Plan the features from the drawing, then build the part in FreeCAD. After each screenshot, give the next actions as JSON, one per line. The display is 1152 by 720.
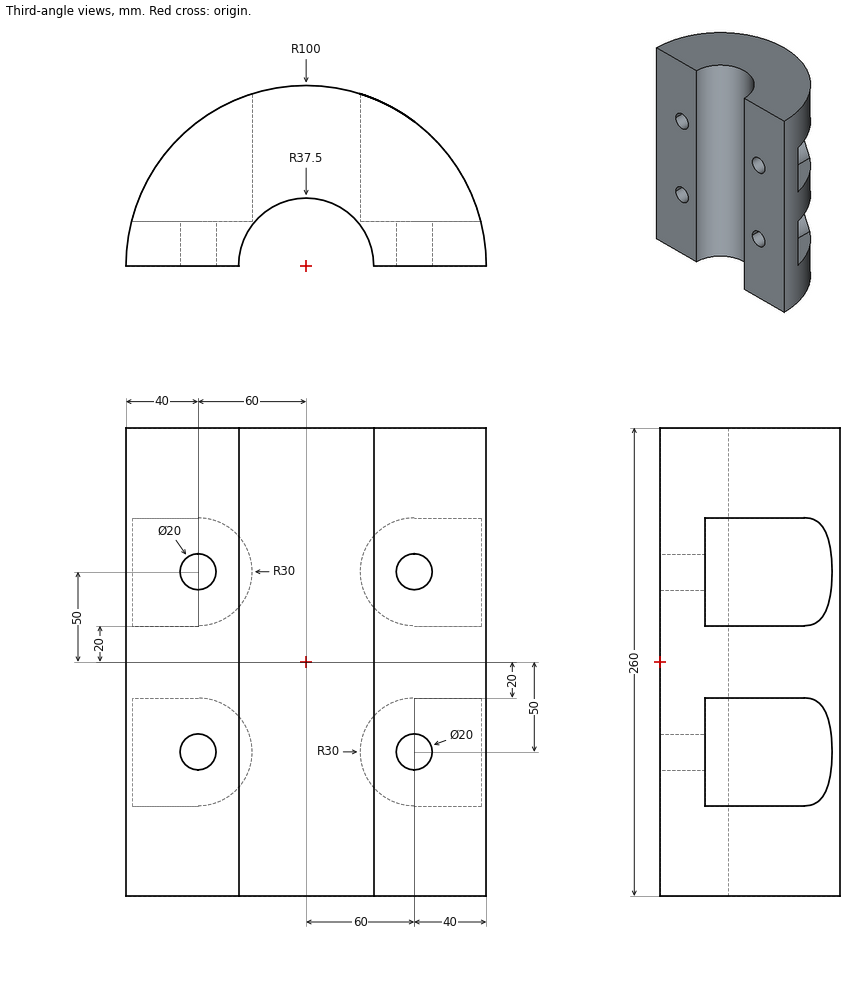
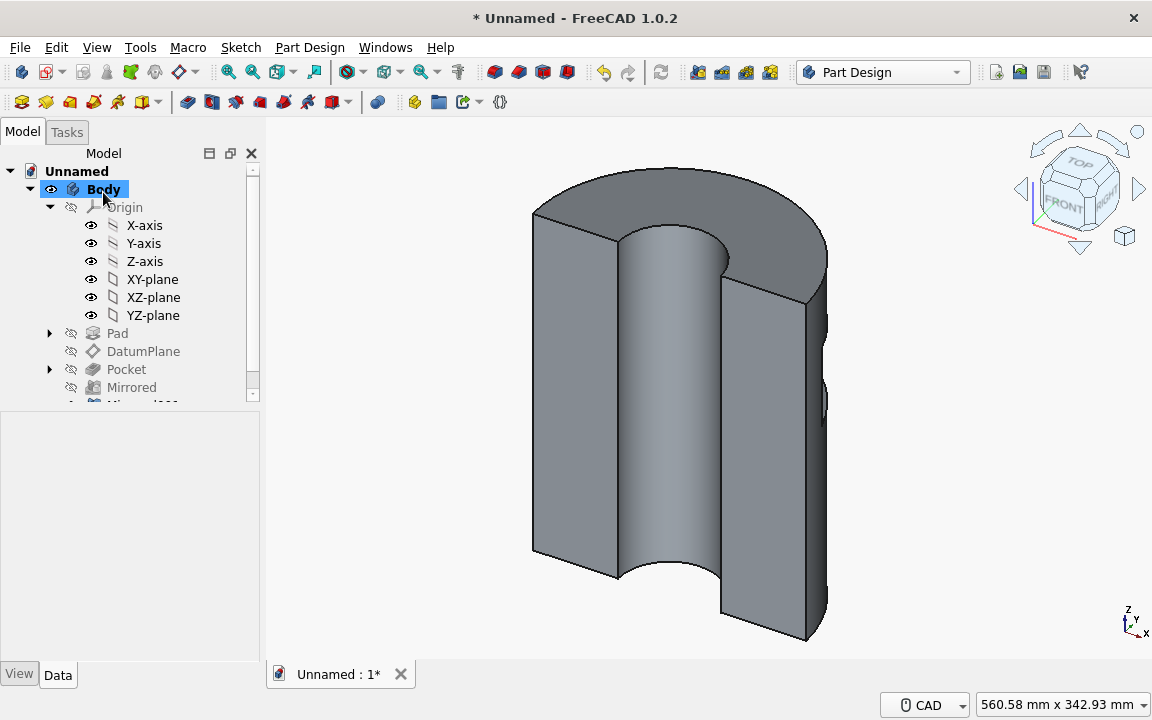
{"action": "key", "text": "4"}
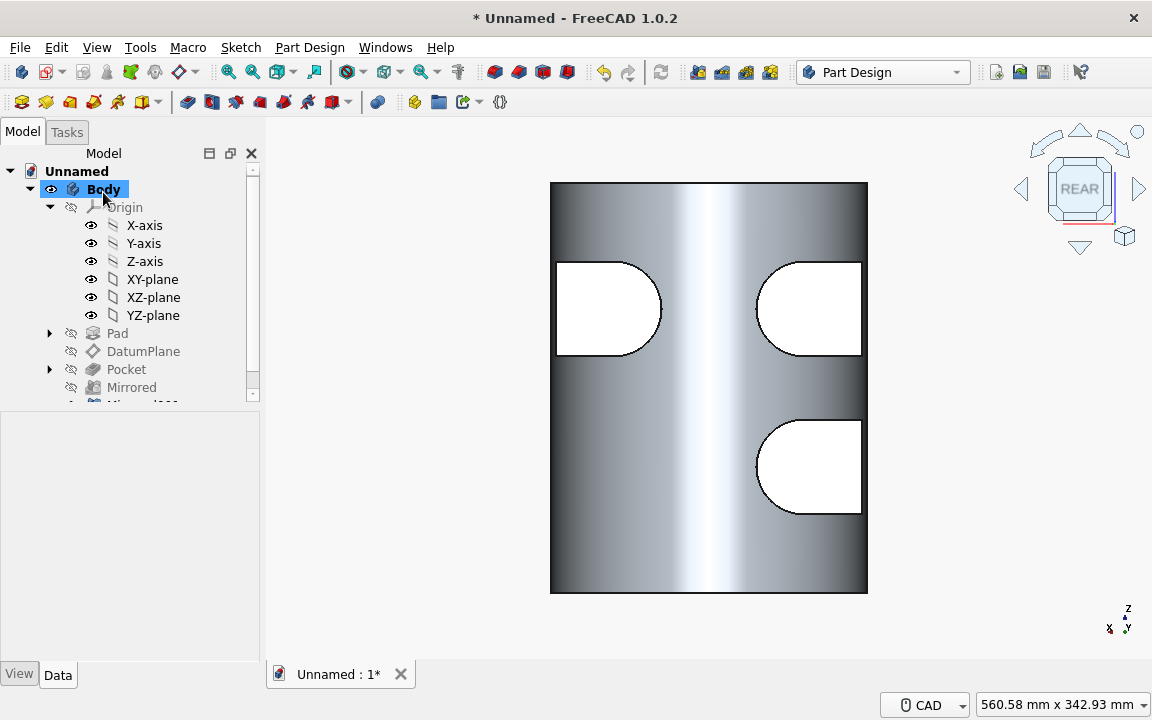
{"action": "left_click", "coordinate": [609, 308]}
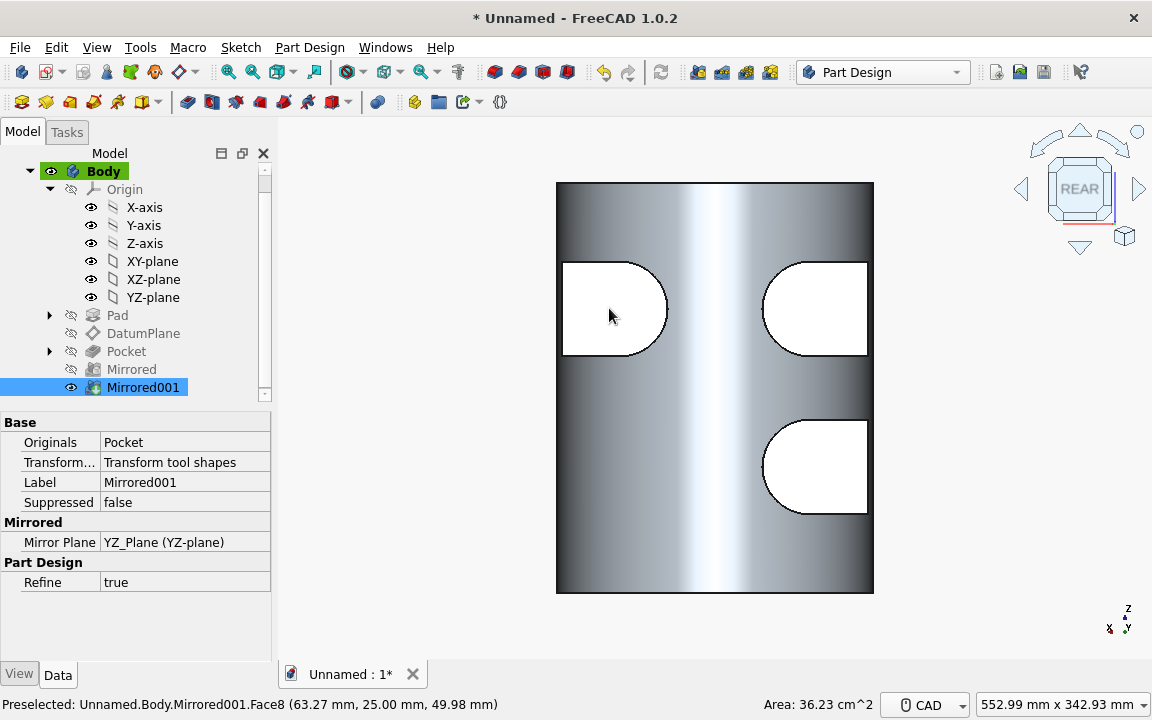
{"action": "left_click", "coordinate": [46, 72]}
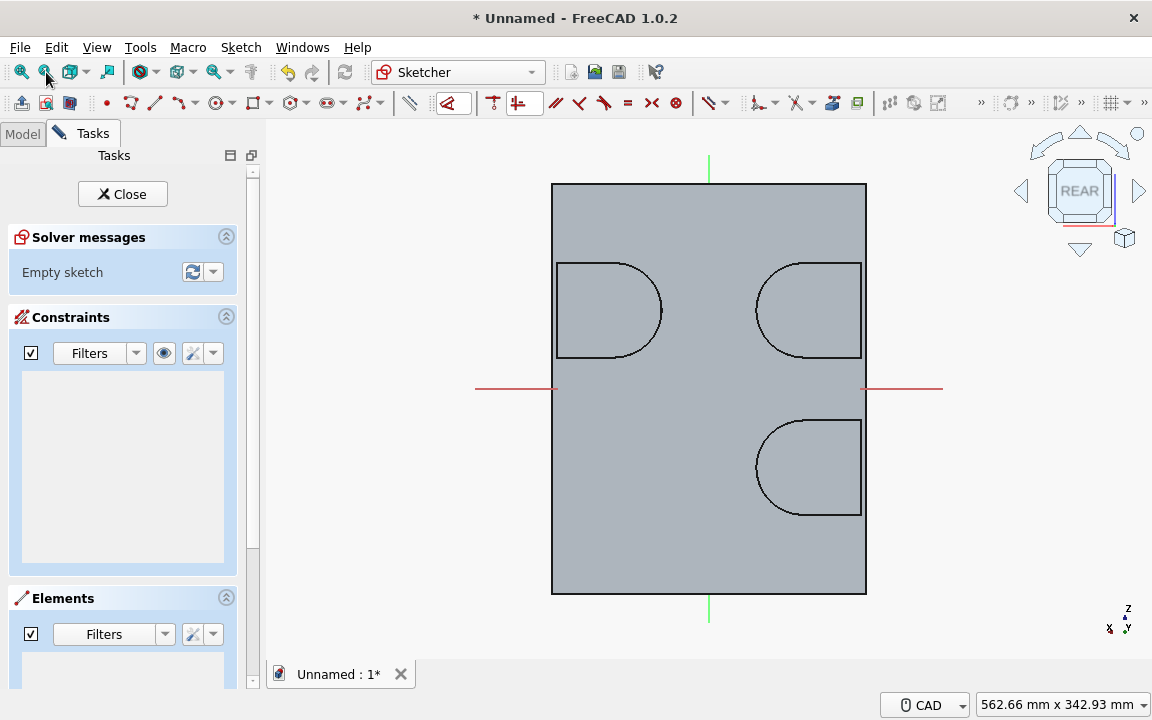
{"action": "scroll", "coordinate": [624, 489], "scroll_direction": "up", "scroll_amount": 5}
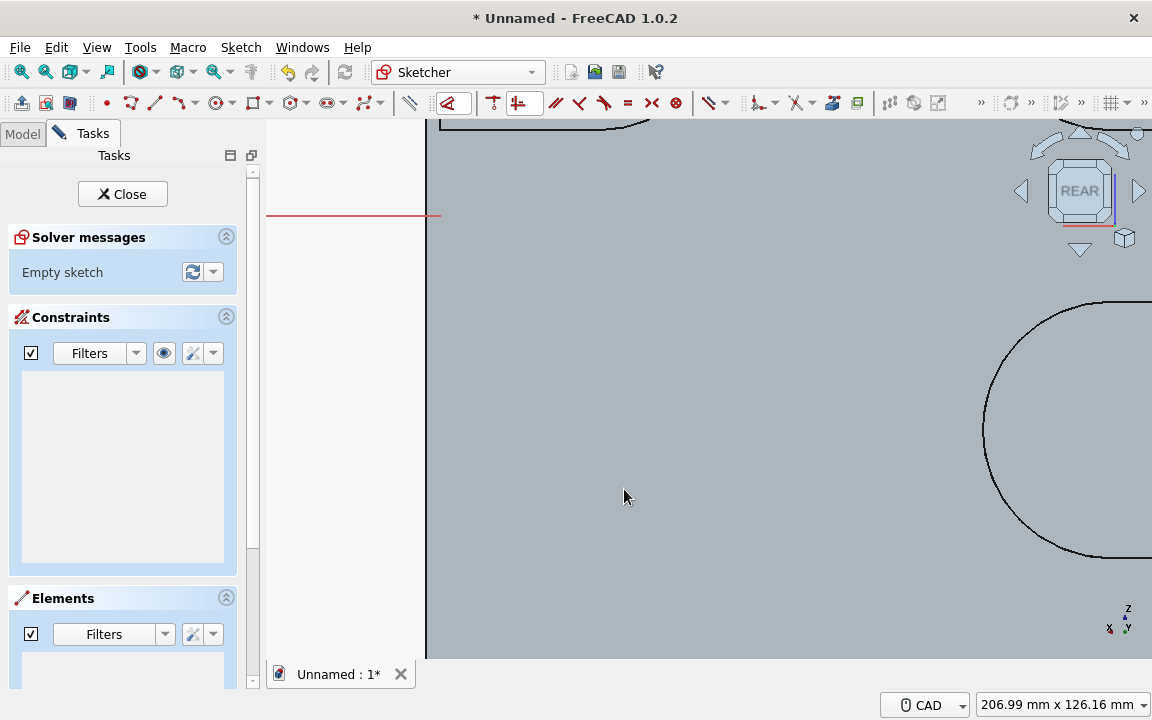
{"action": "left_click", "coordinate": [132, 104]}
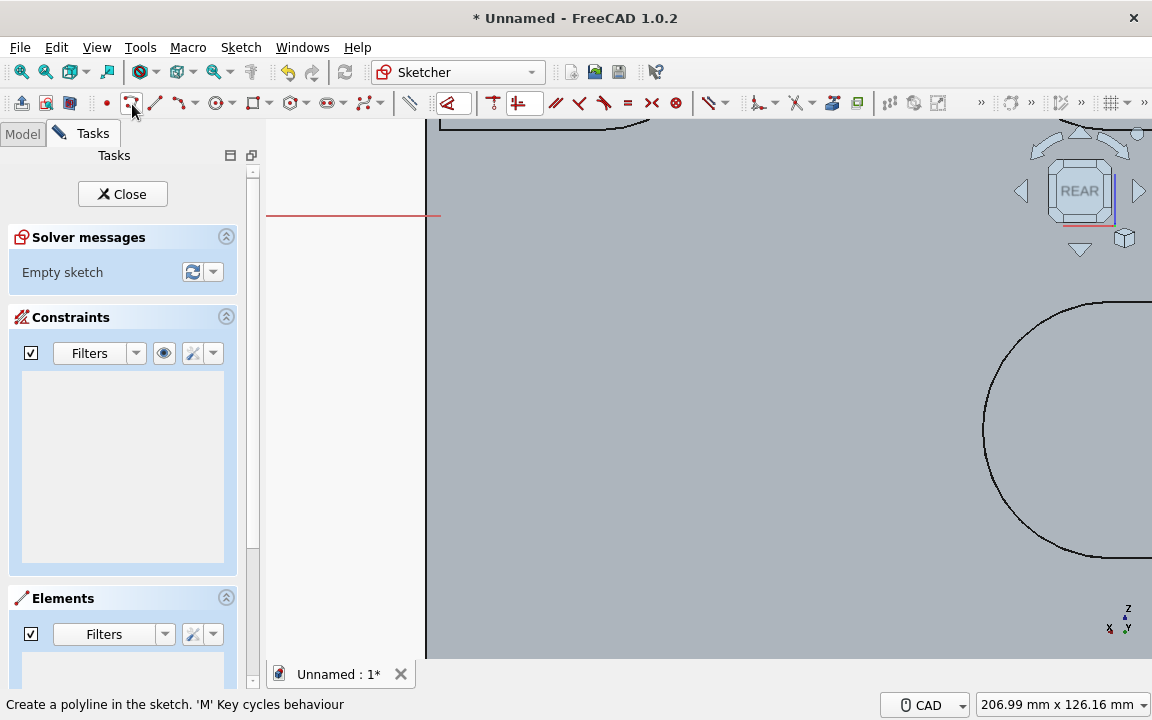
{"action": "left_click", "coordinate": [598, 302]}
{"action": "left_click", "coordinate": [426, 302]}
{"action": "left_click", "coordinate": [426, 558]}
{"action": "left_click", "coordinate": [598, 558]}
{"action": "right_click", "coordinate": [598, 558]}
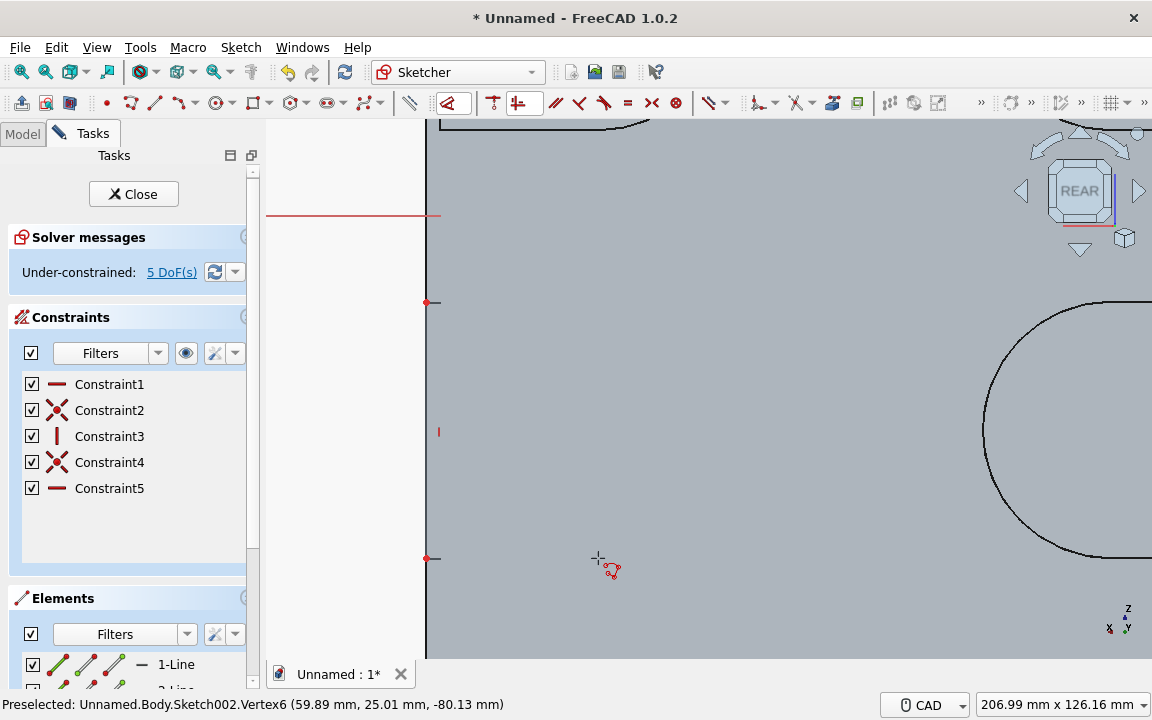
{"action": "key", "text": "g 3 a"}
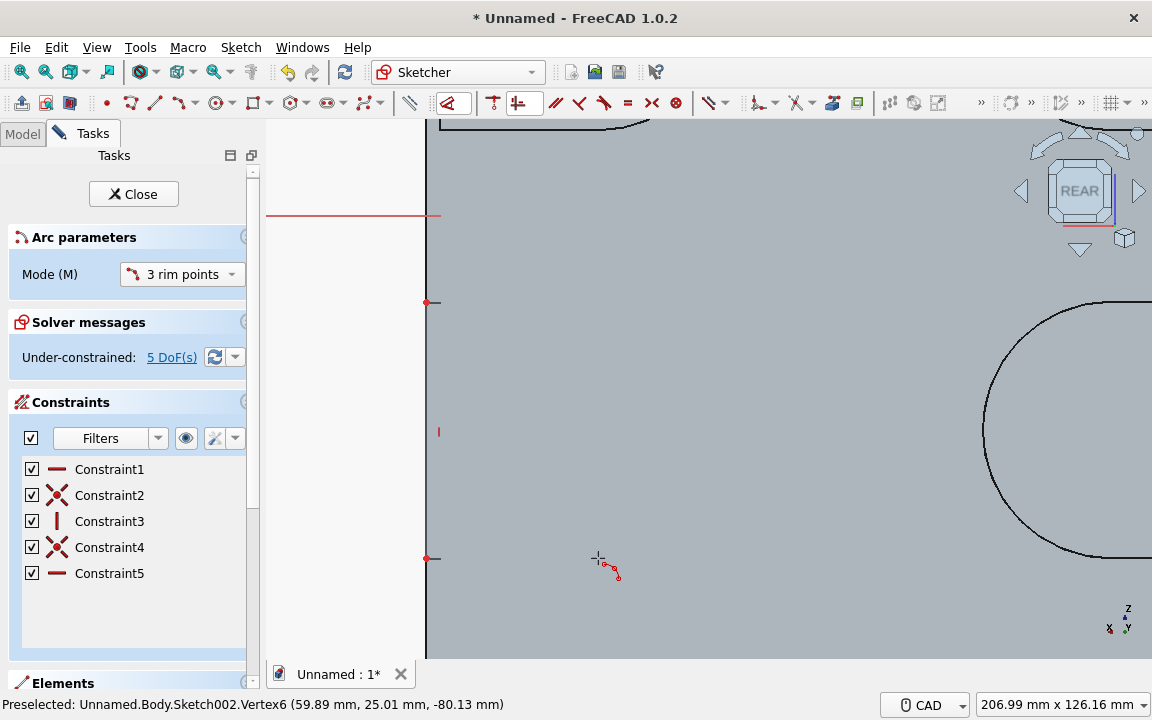
{"action": "left_click", "coordinate": [598, 559]}
{"action": "left_click", "coordinate": [598, 303]}
{"action": "left_click", "coordinate": [726, 430]}
{"action": "key", "text": "Escape"}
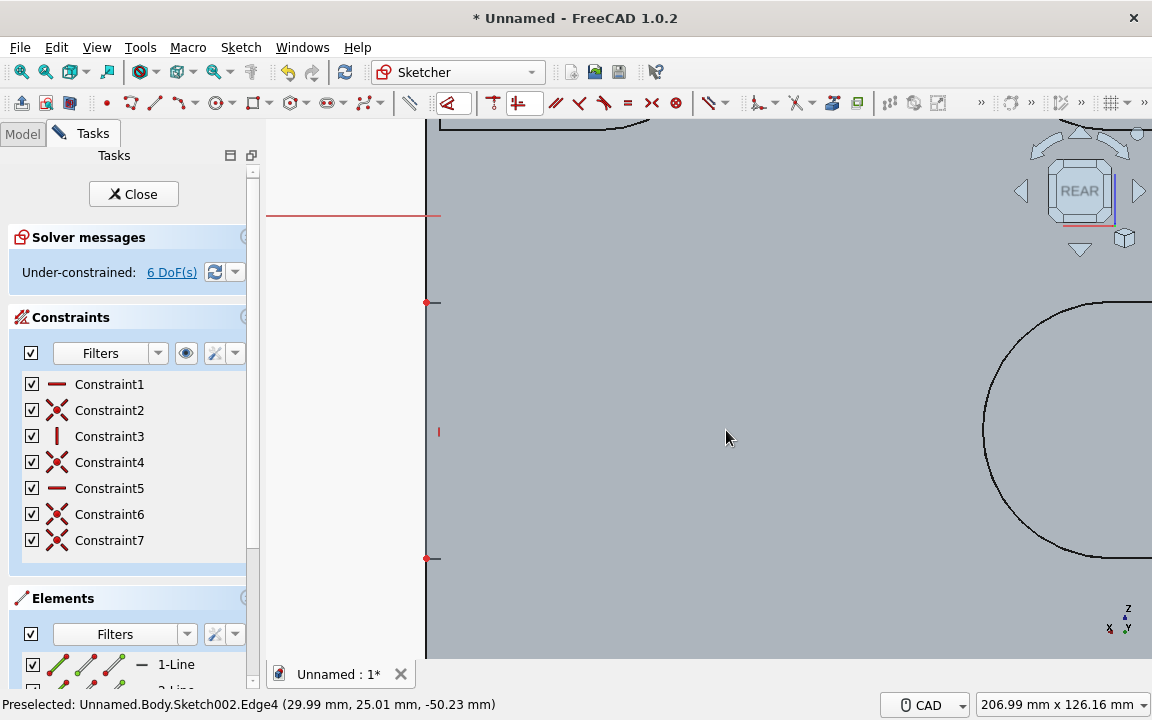
{"action": "left_click", "coordinate": [546, 303]}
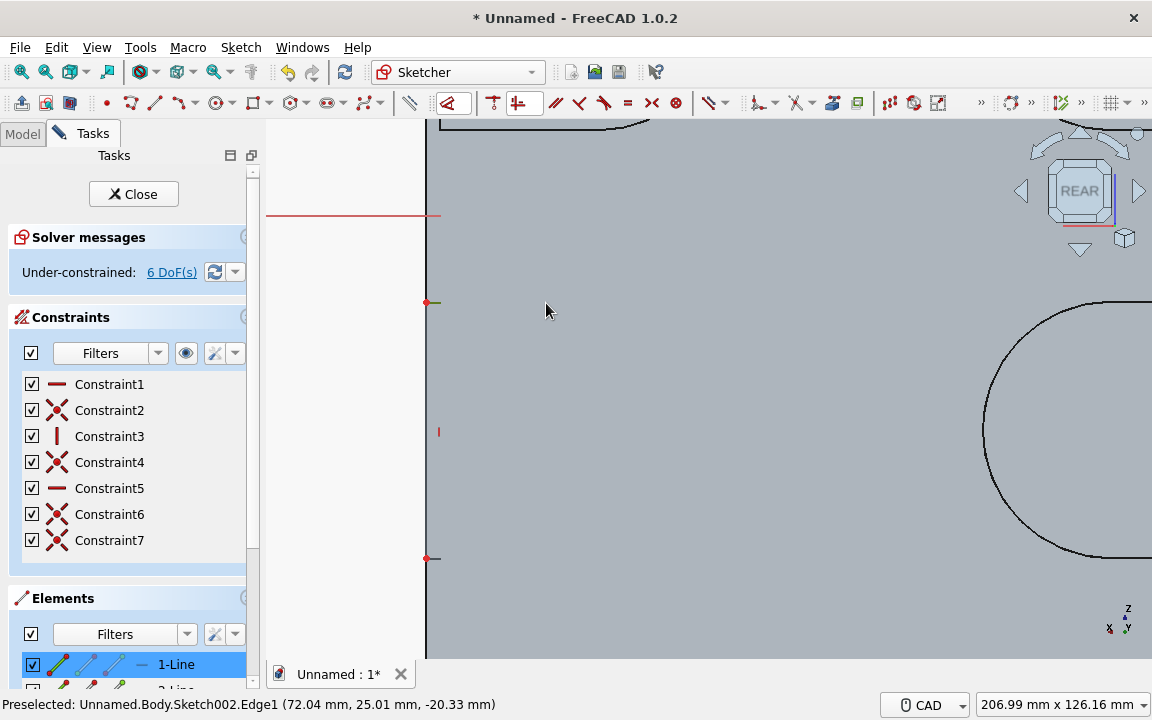
{"action": "left_click", "coordinate": [702, 506]}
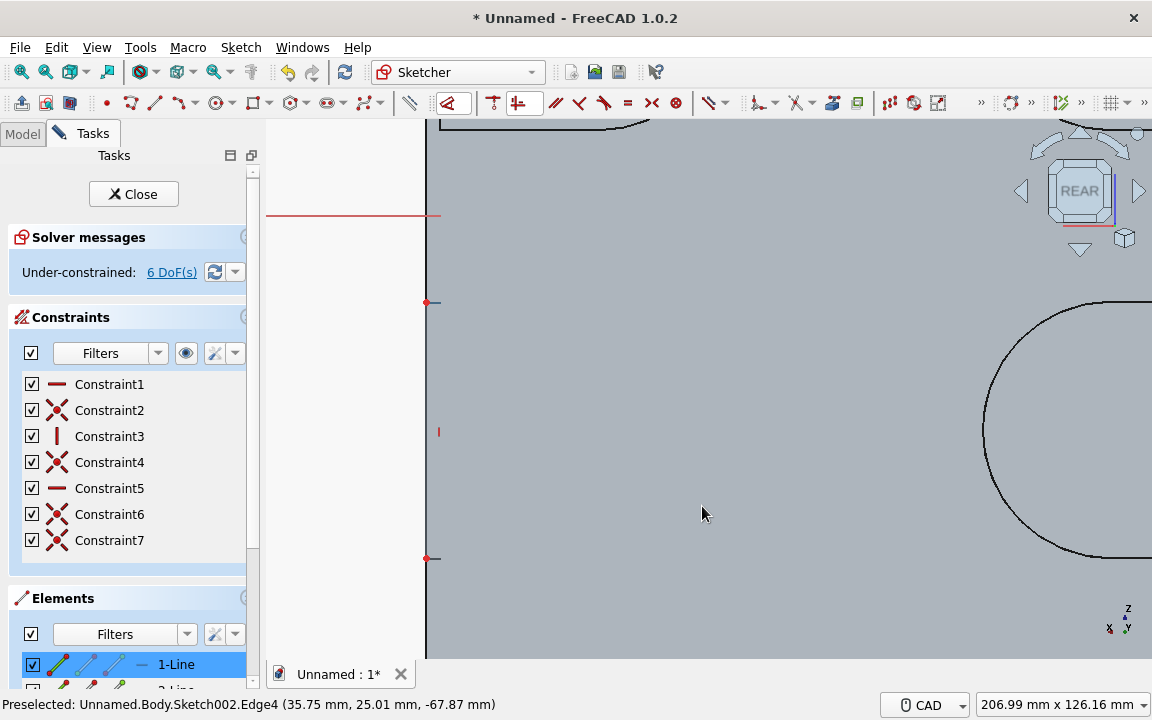
{"action": "key", "text": "t"}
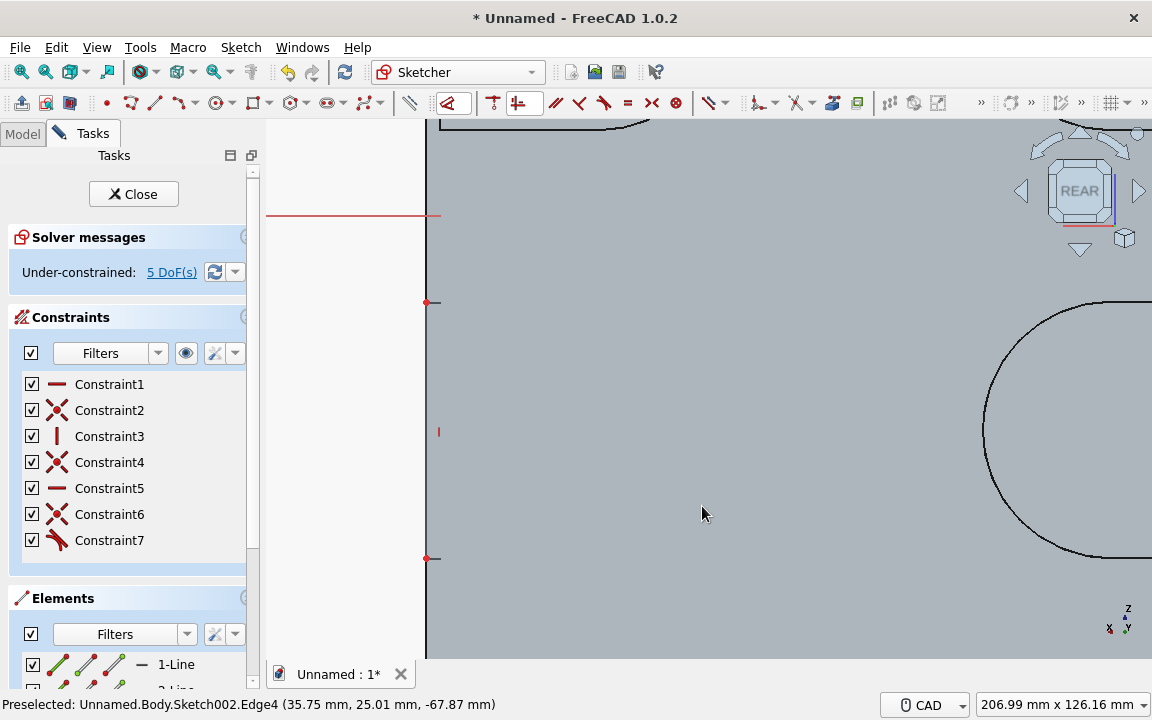
{"action": "left_click", "coordinate": [478, 559]}